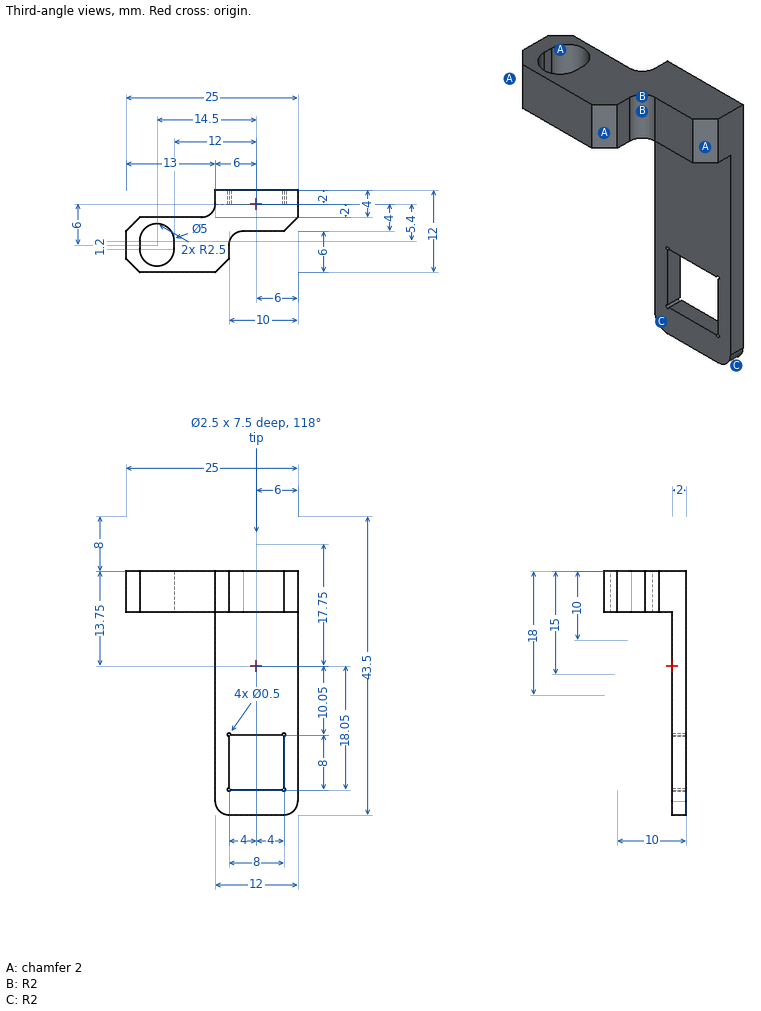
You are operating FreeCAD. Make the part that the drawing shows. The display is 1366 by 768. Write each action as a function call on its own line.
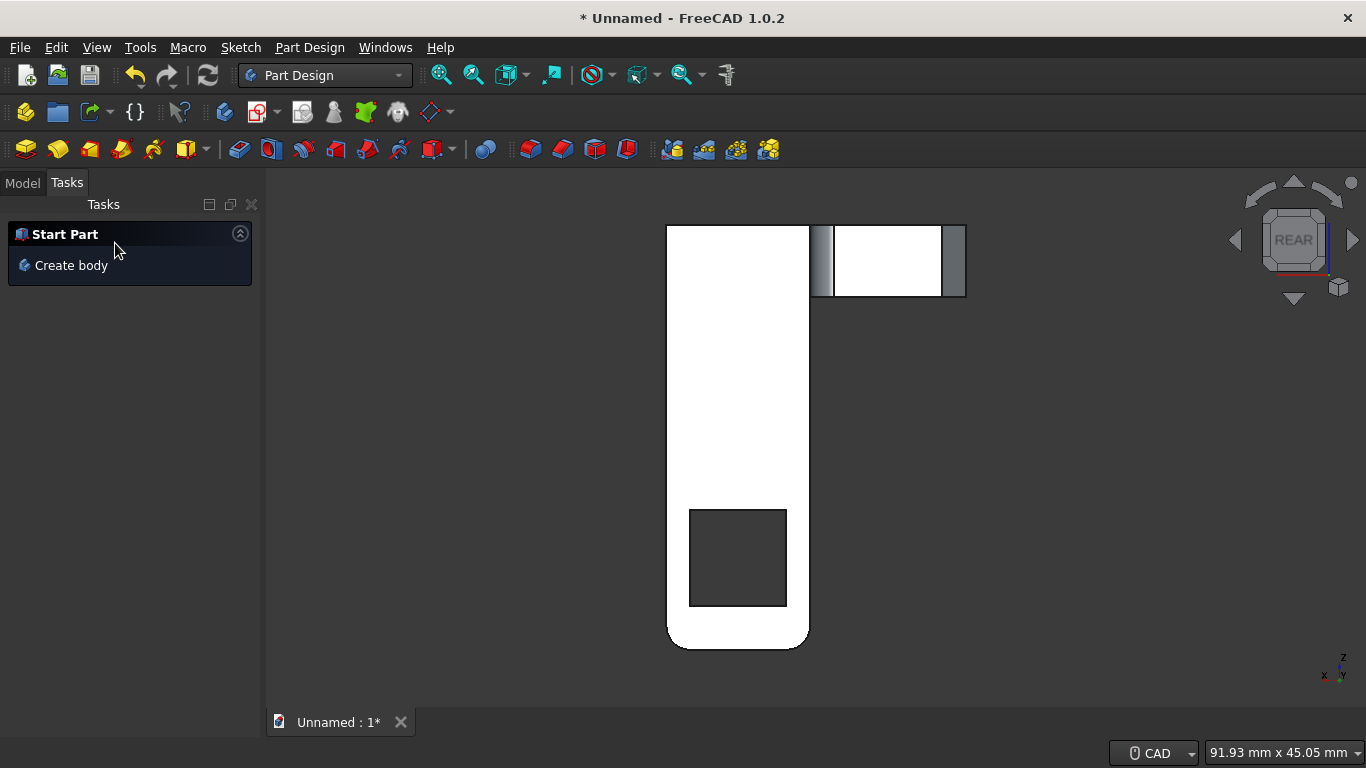
click(738, 315)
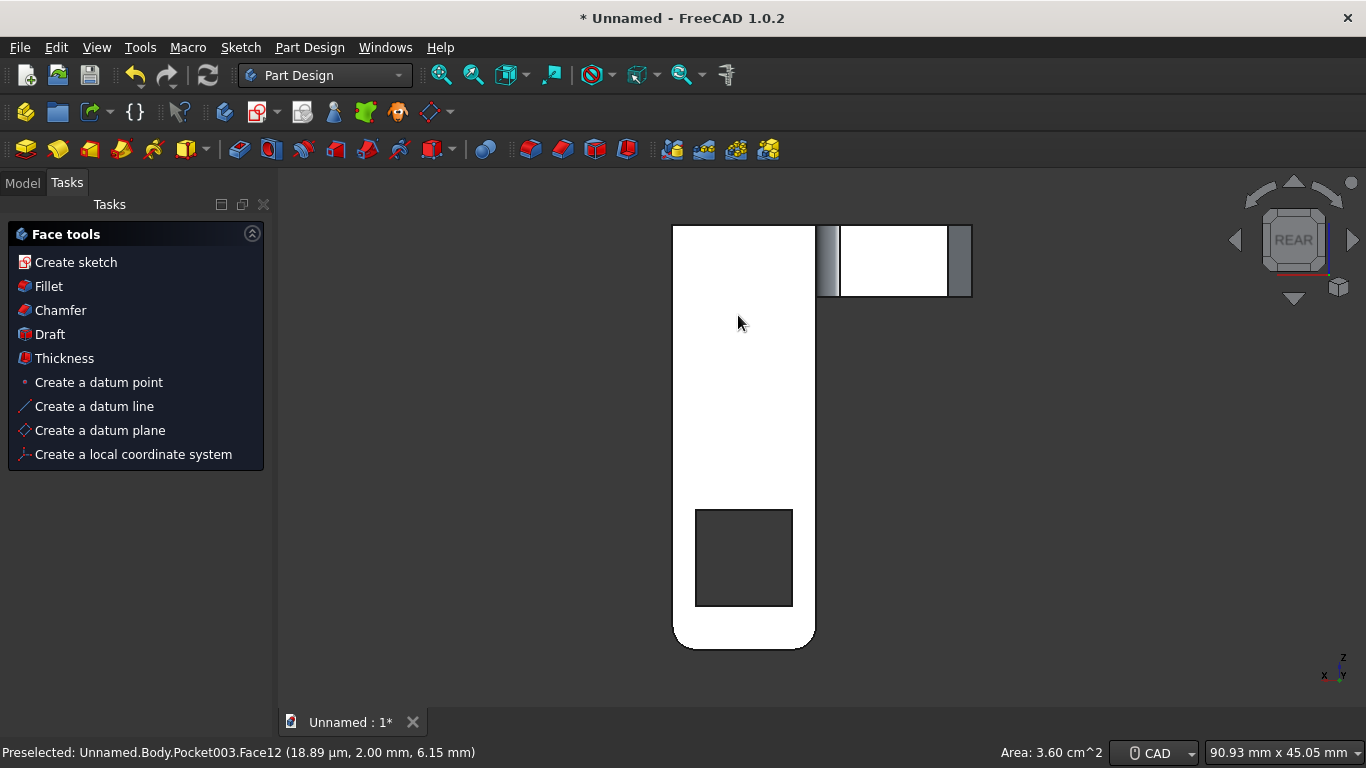
click(258, 112)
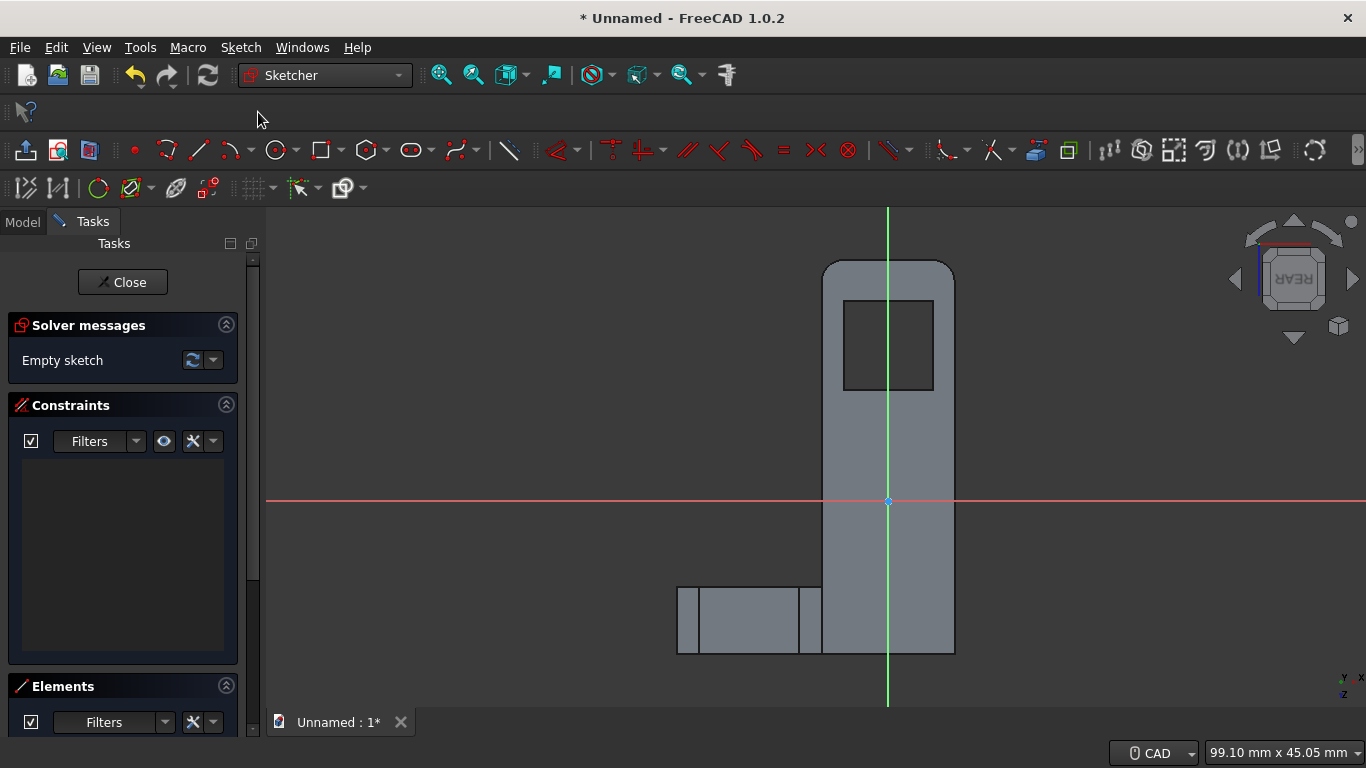
scroll(1174, 284, up, 2)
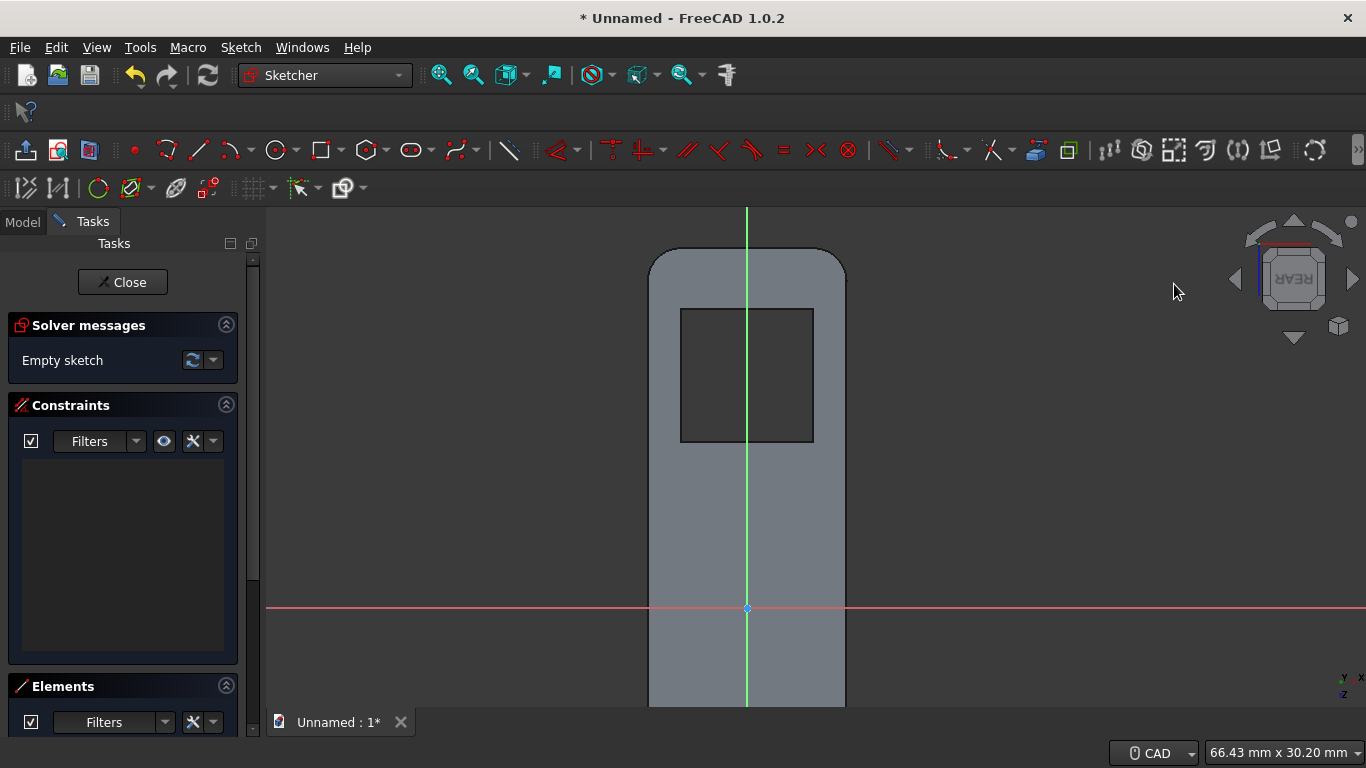
click(276, 150)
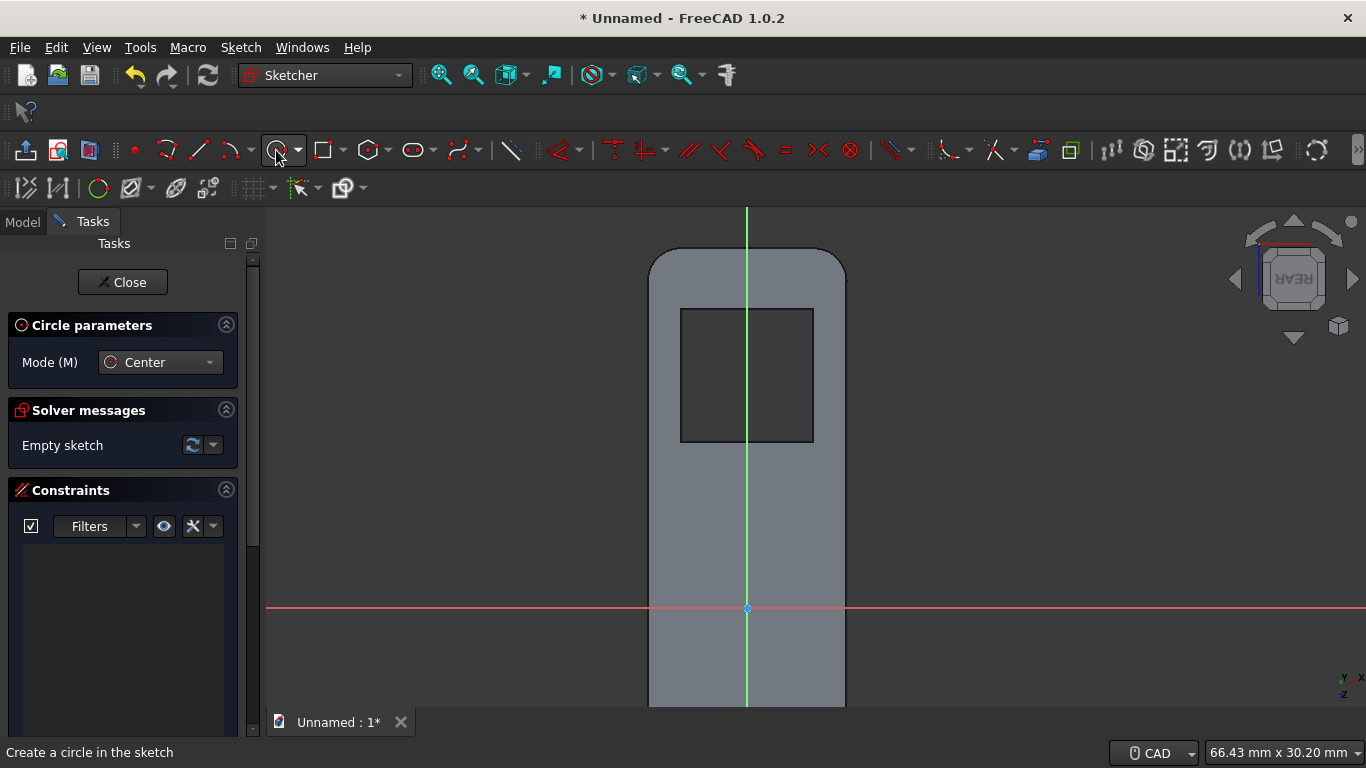
scroll(681, 442, up, 9)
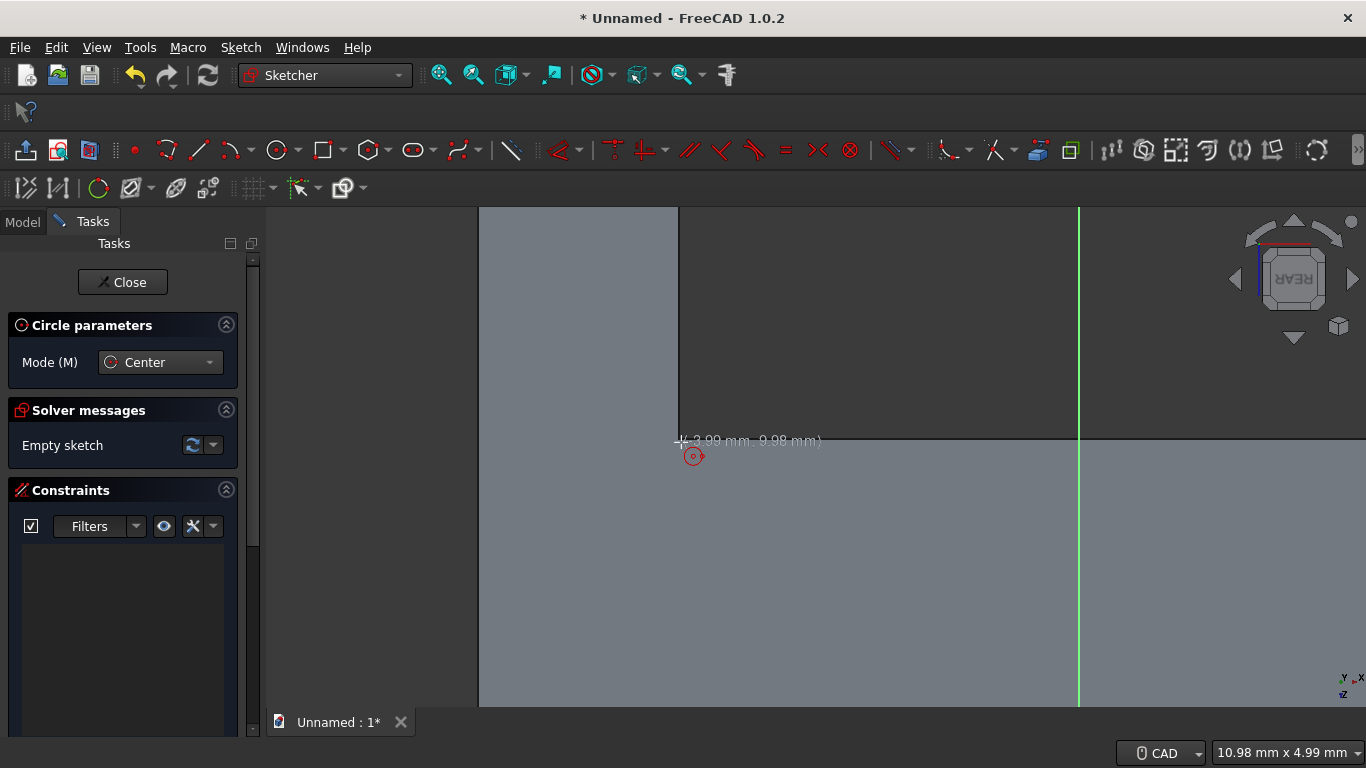
scroll(682, 443, down, 9)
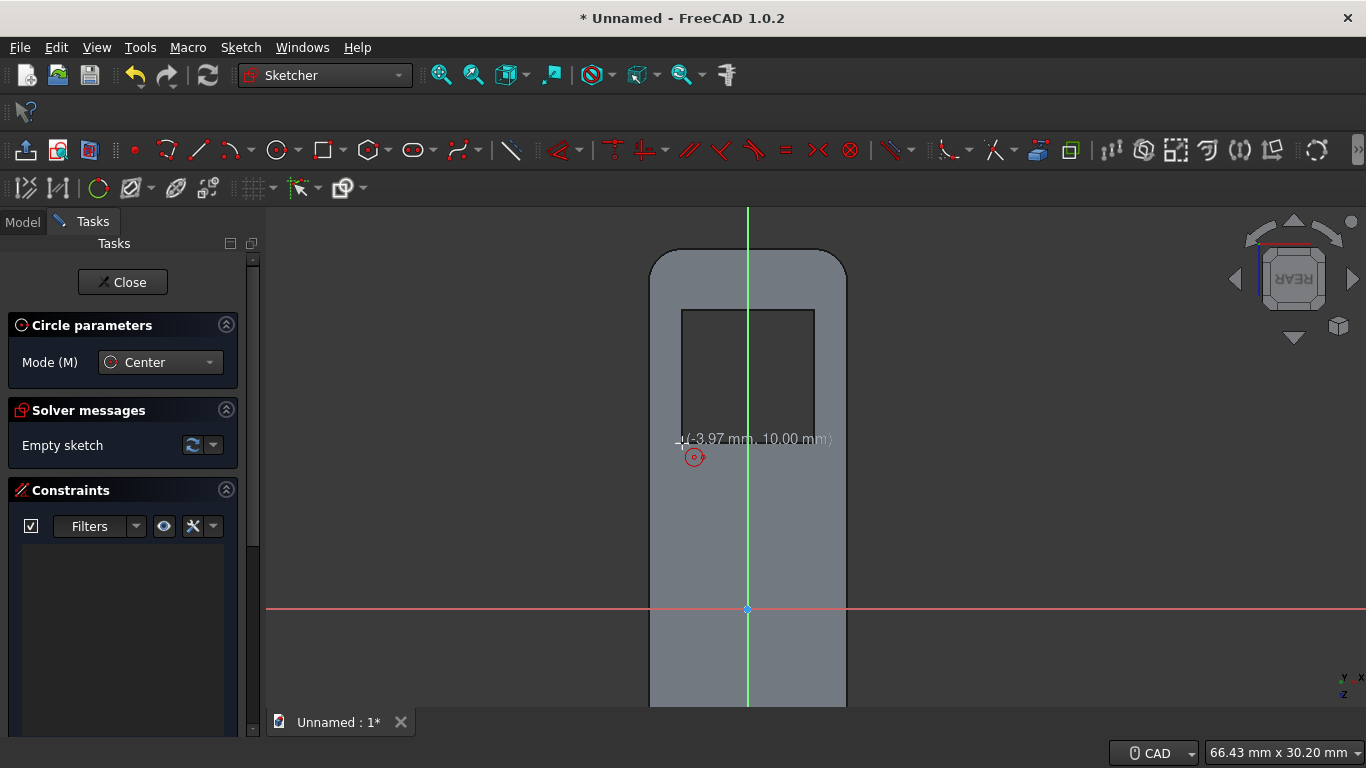
click(682, 443)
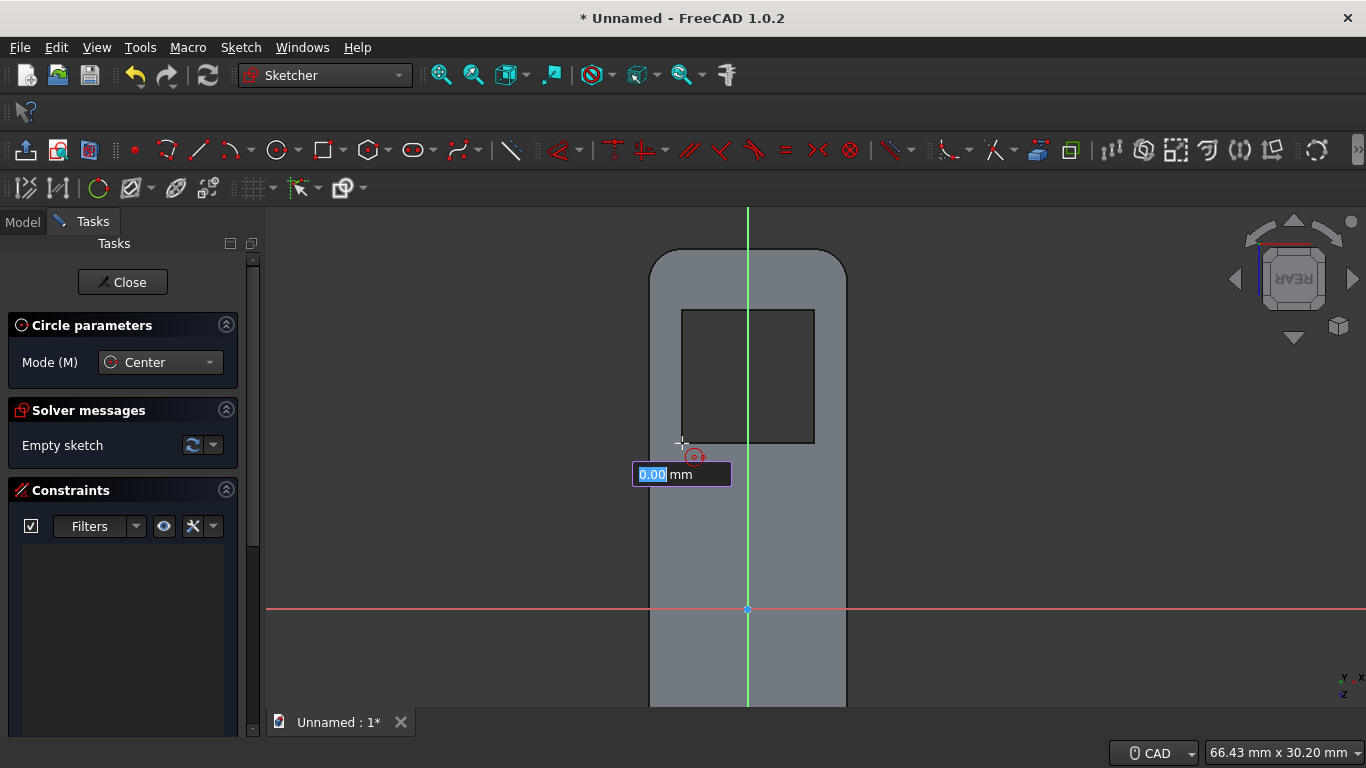
scroll(685, 440, up, 7)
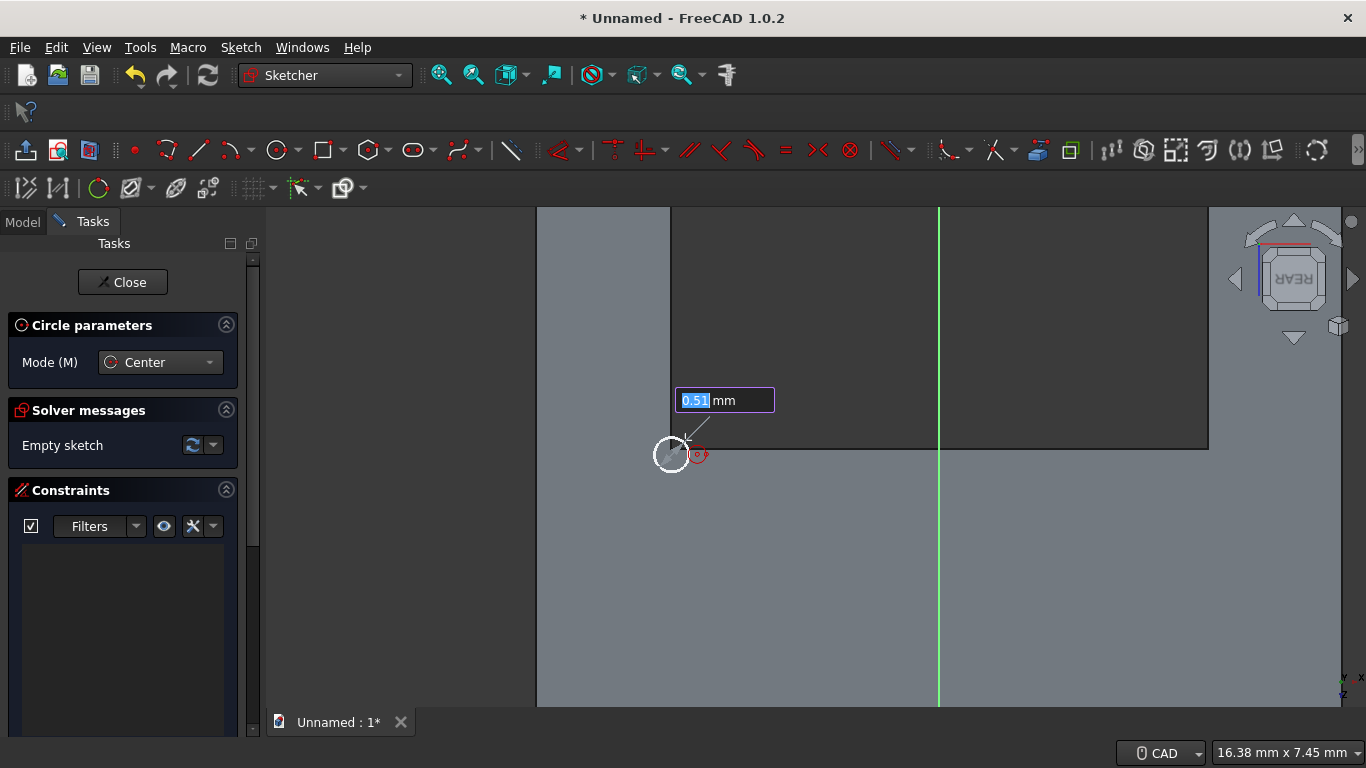
click(683, 438)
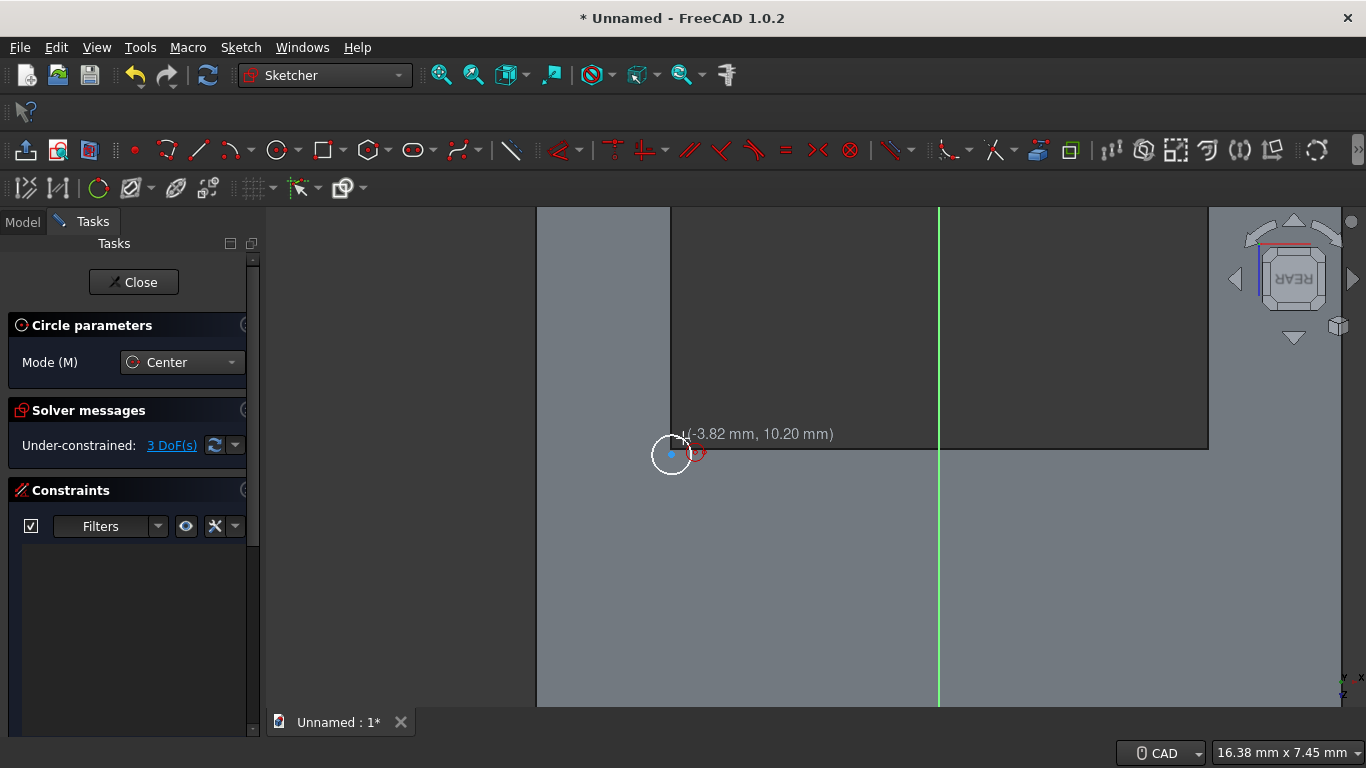
scroll(685, 440, down, 7)